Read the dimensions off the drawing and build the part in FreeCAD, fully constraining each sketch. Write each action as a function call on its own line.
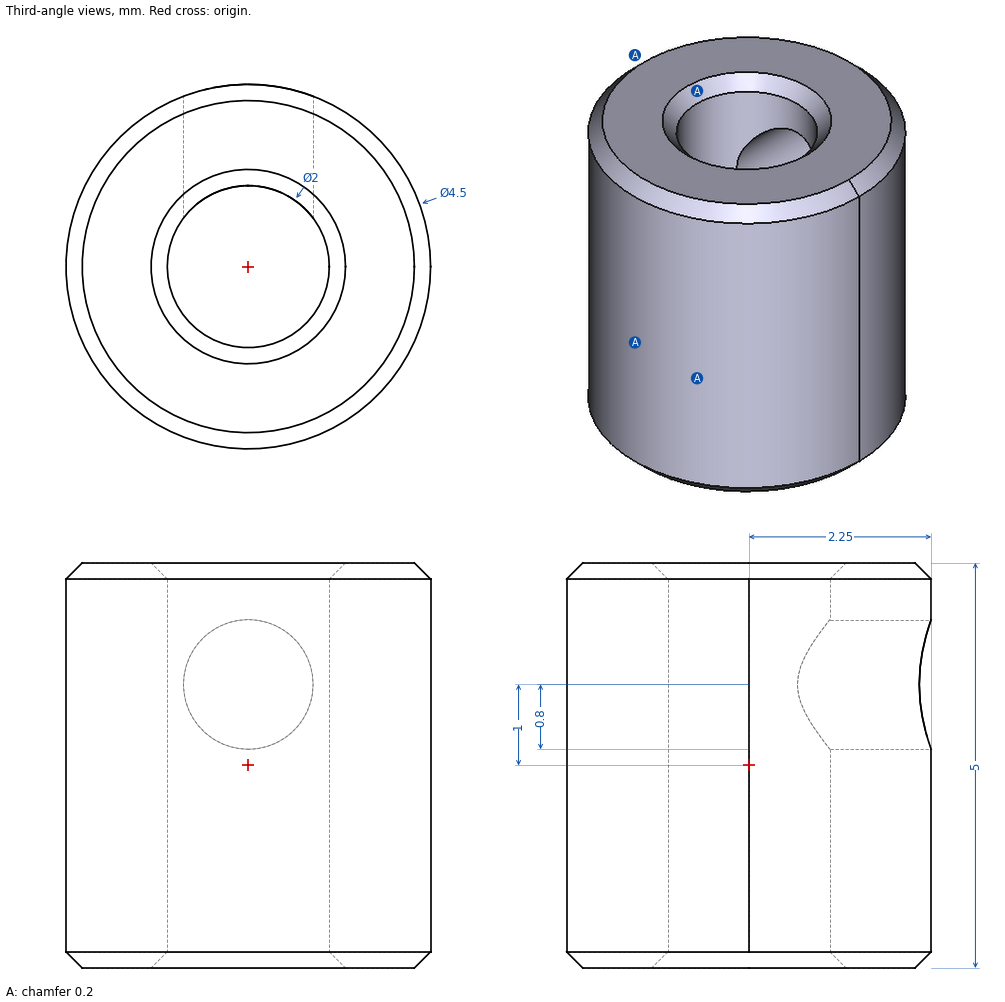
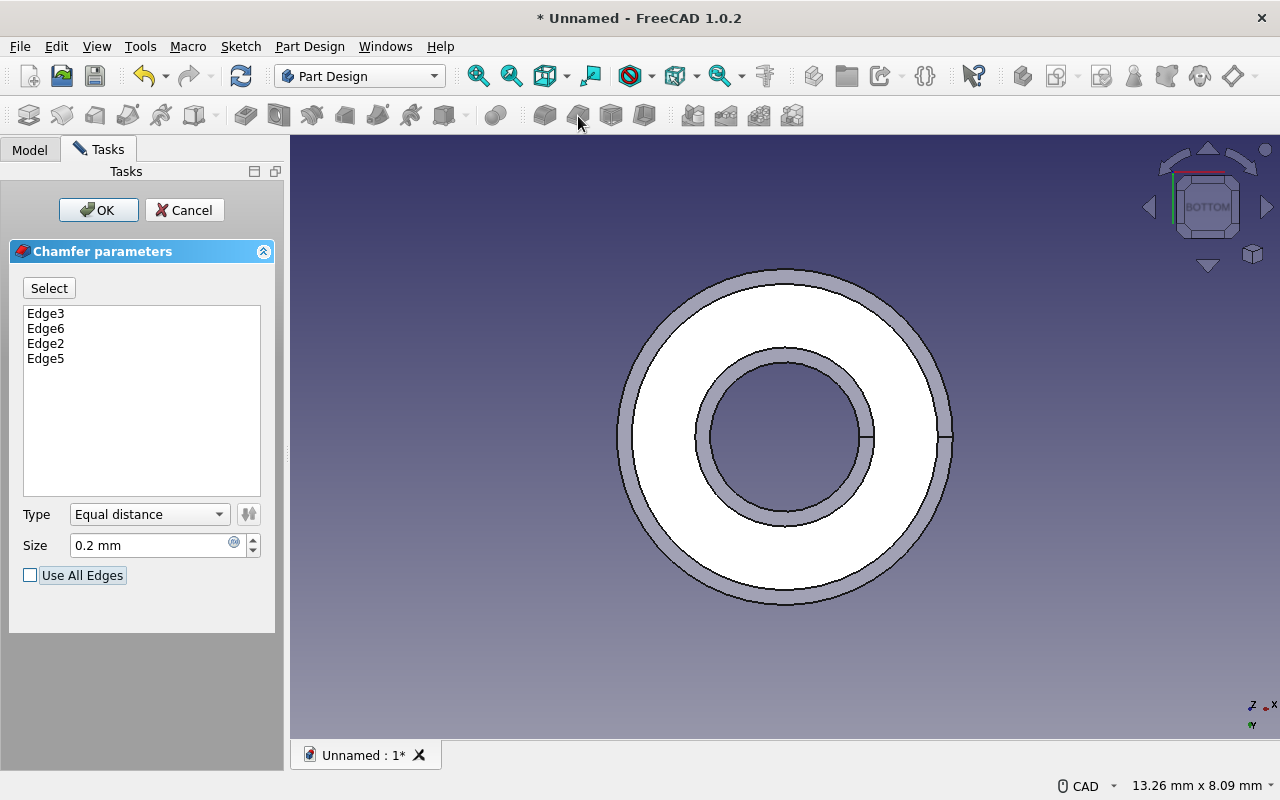
click(99, 210)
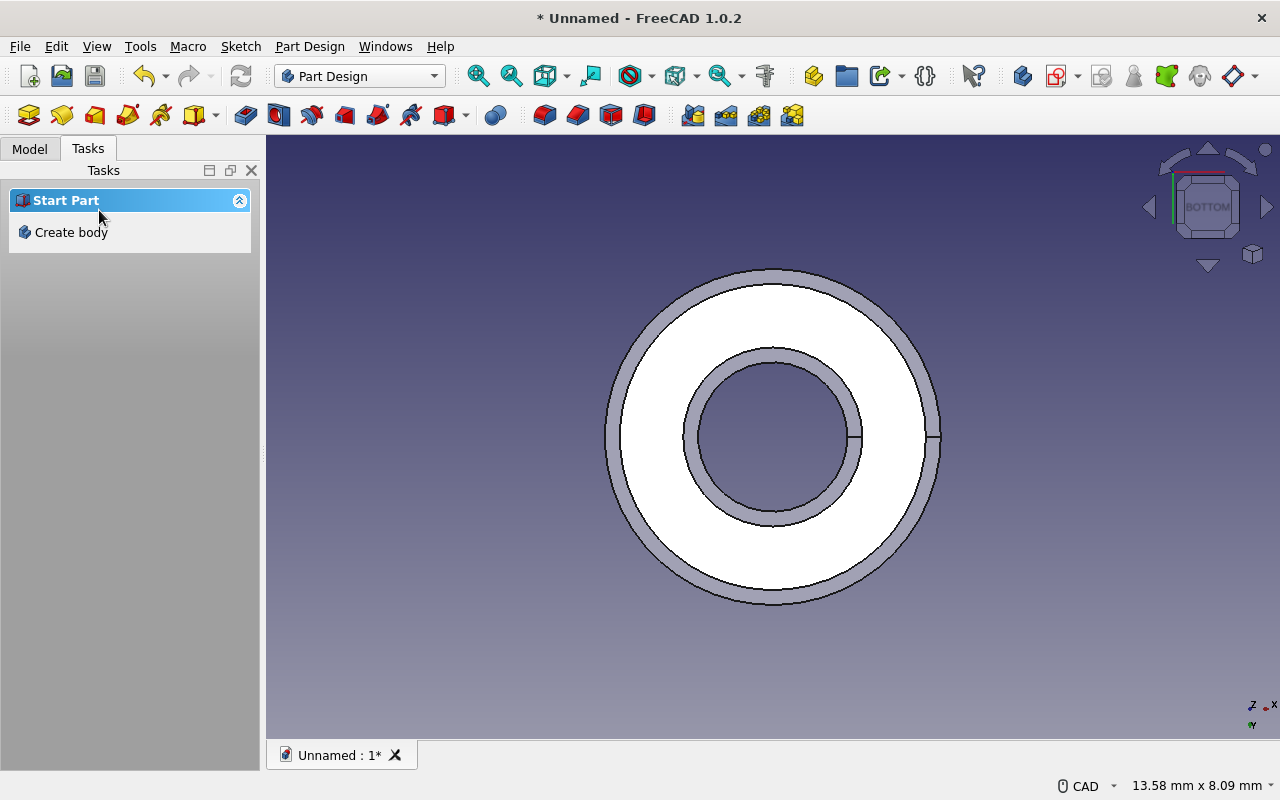
click(1056, 76)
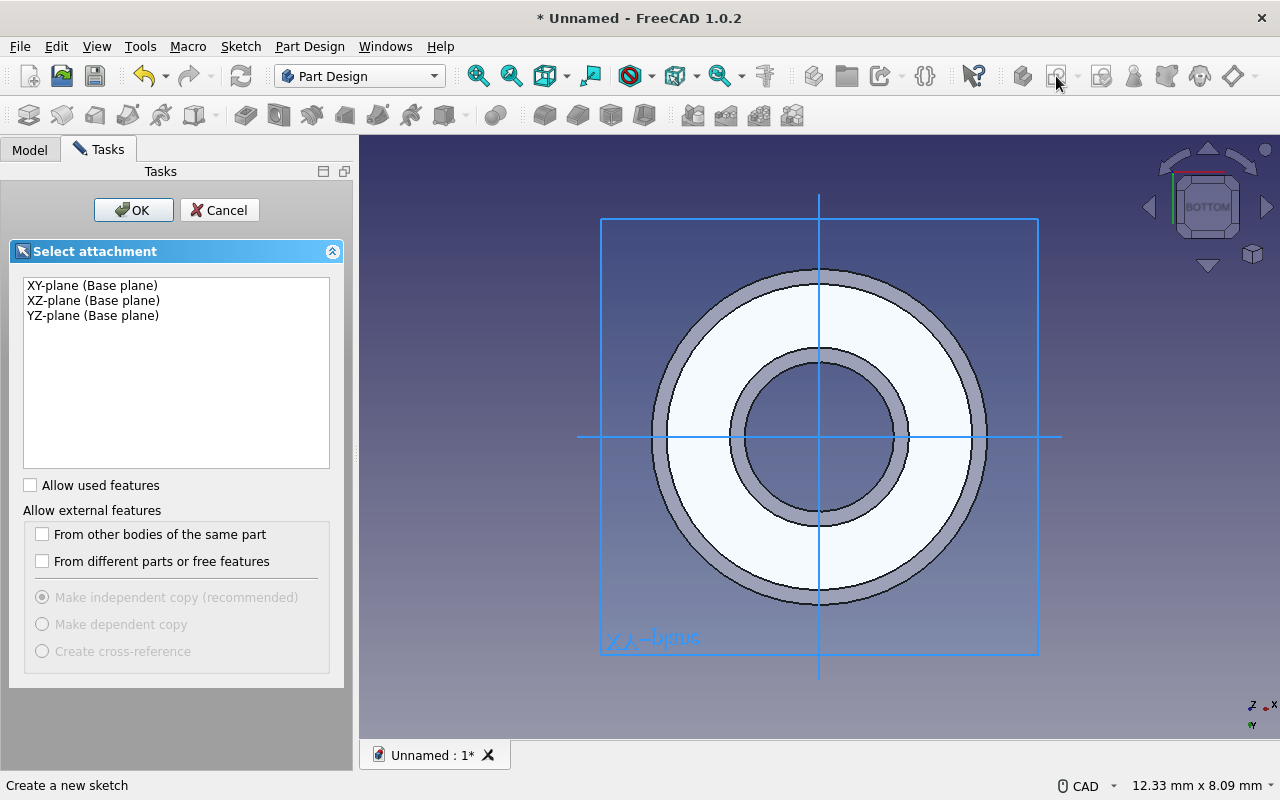
click(84, 316)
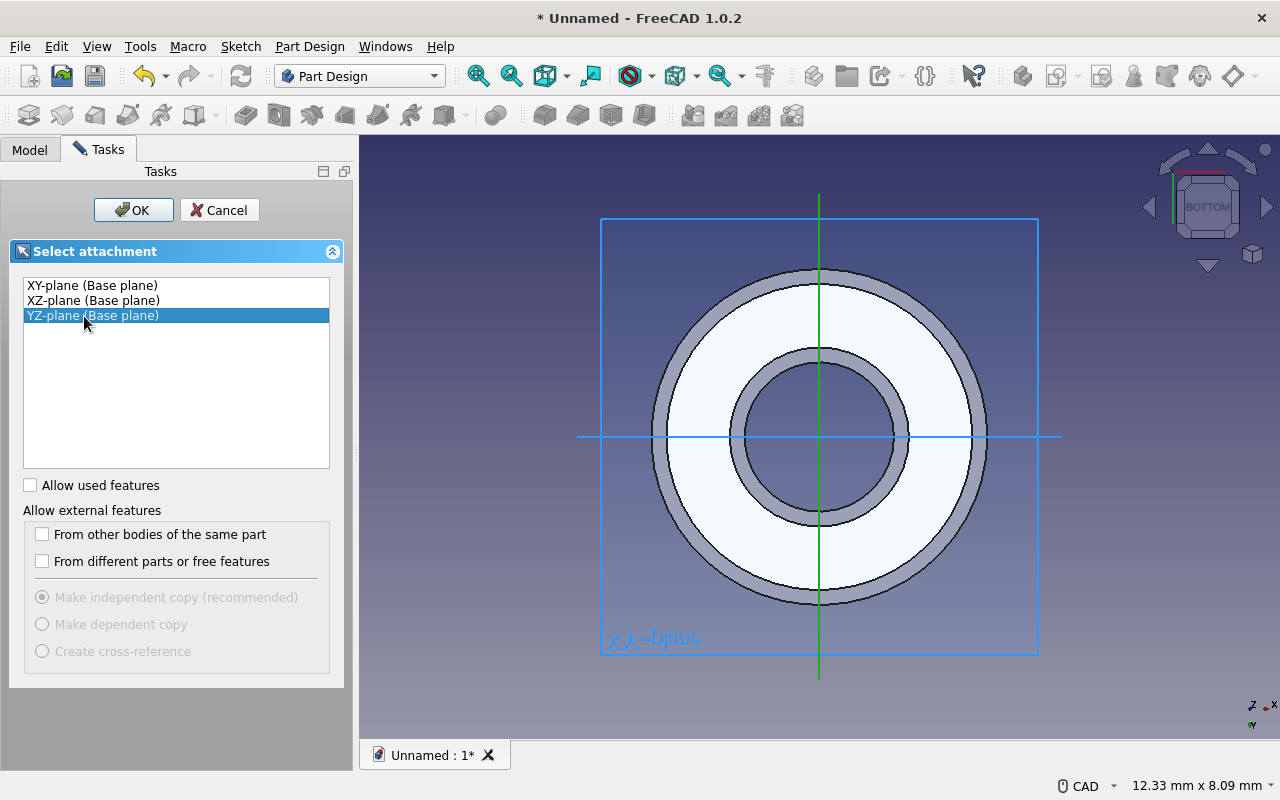
click(134, 210)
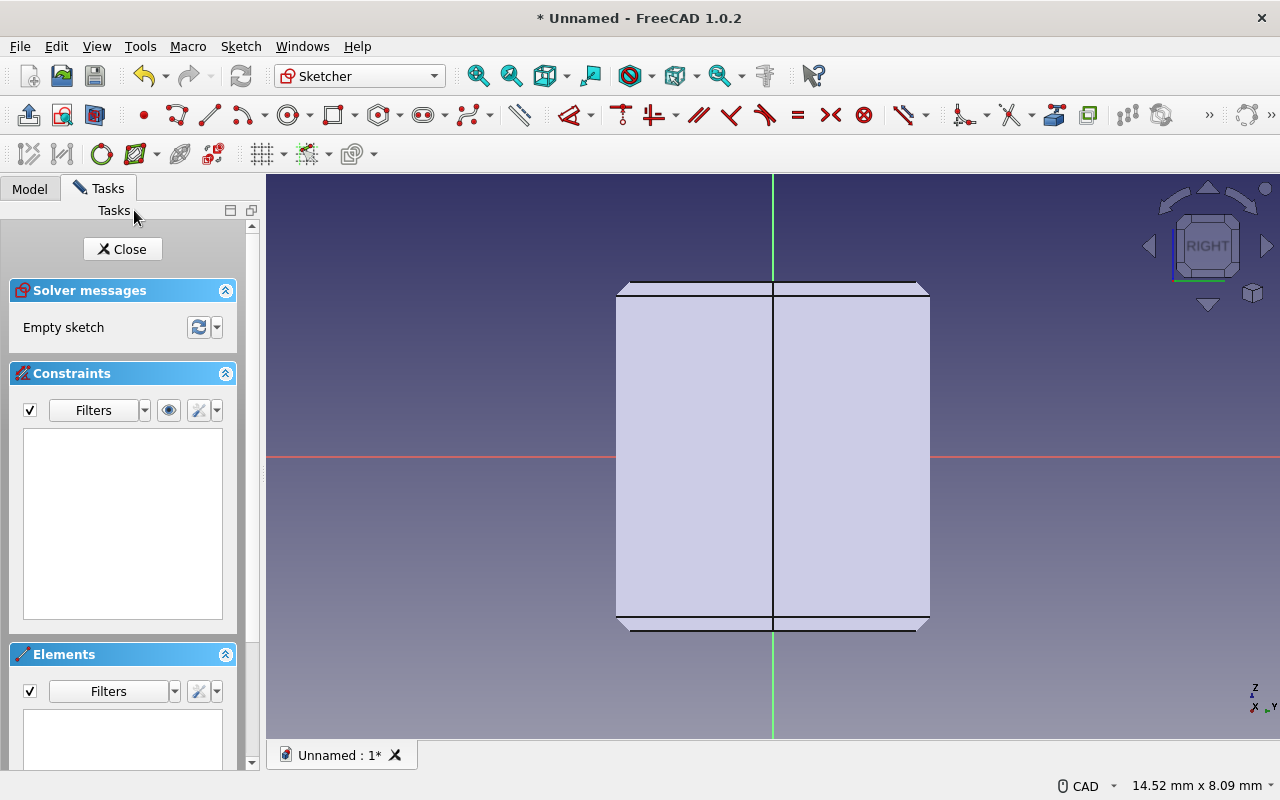
click(95, 116)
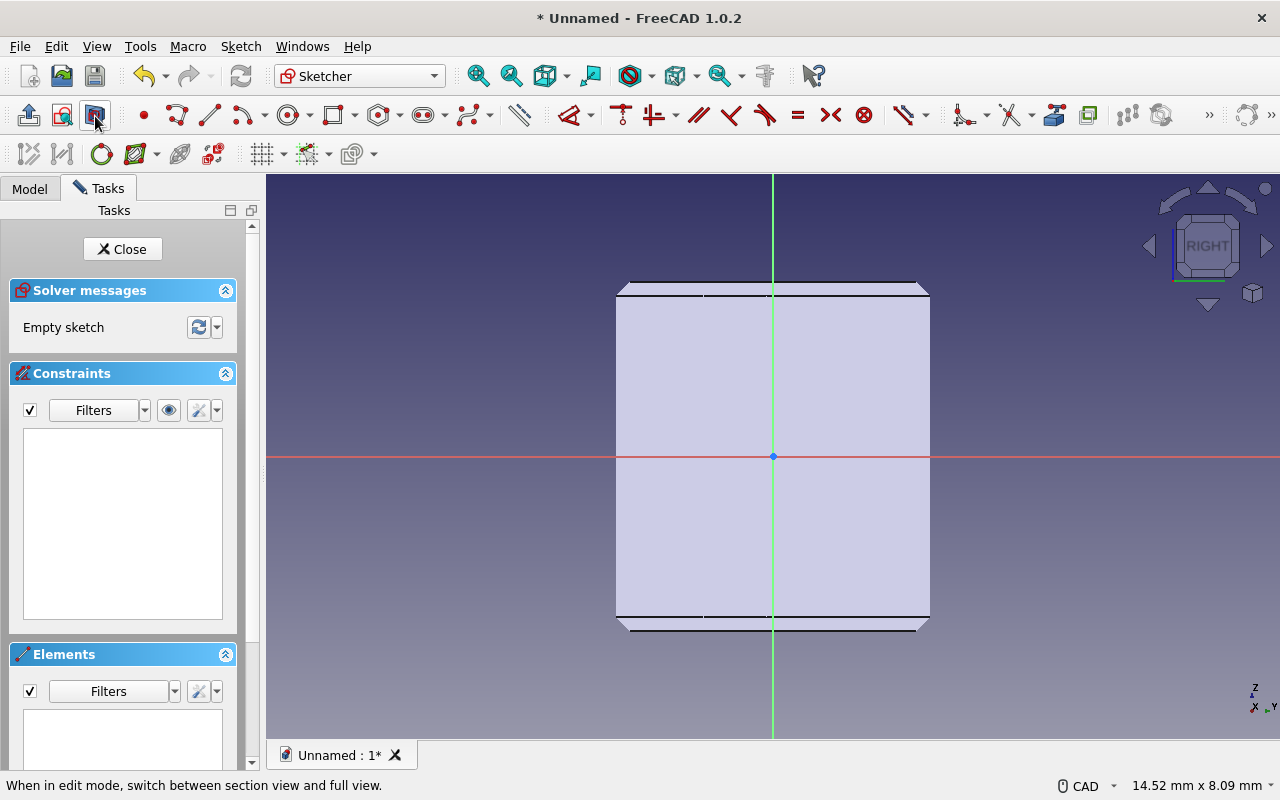
scroll(987, 401, up, 5)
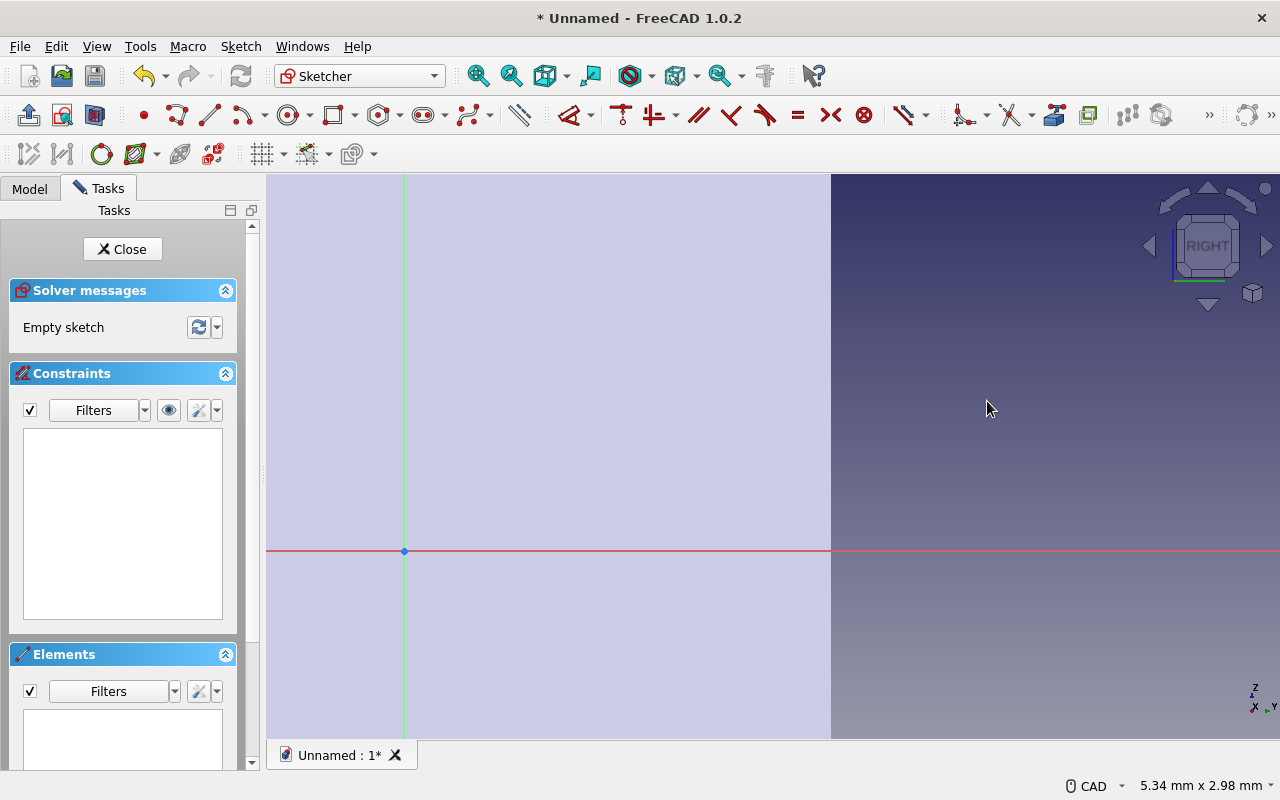
key(g)
key(r)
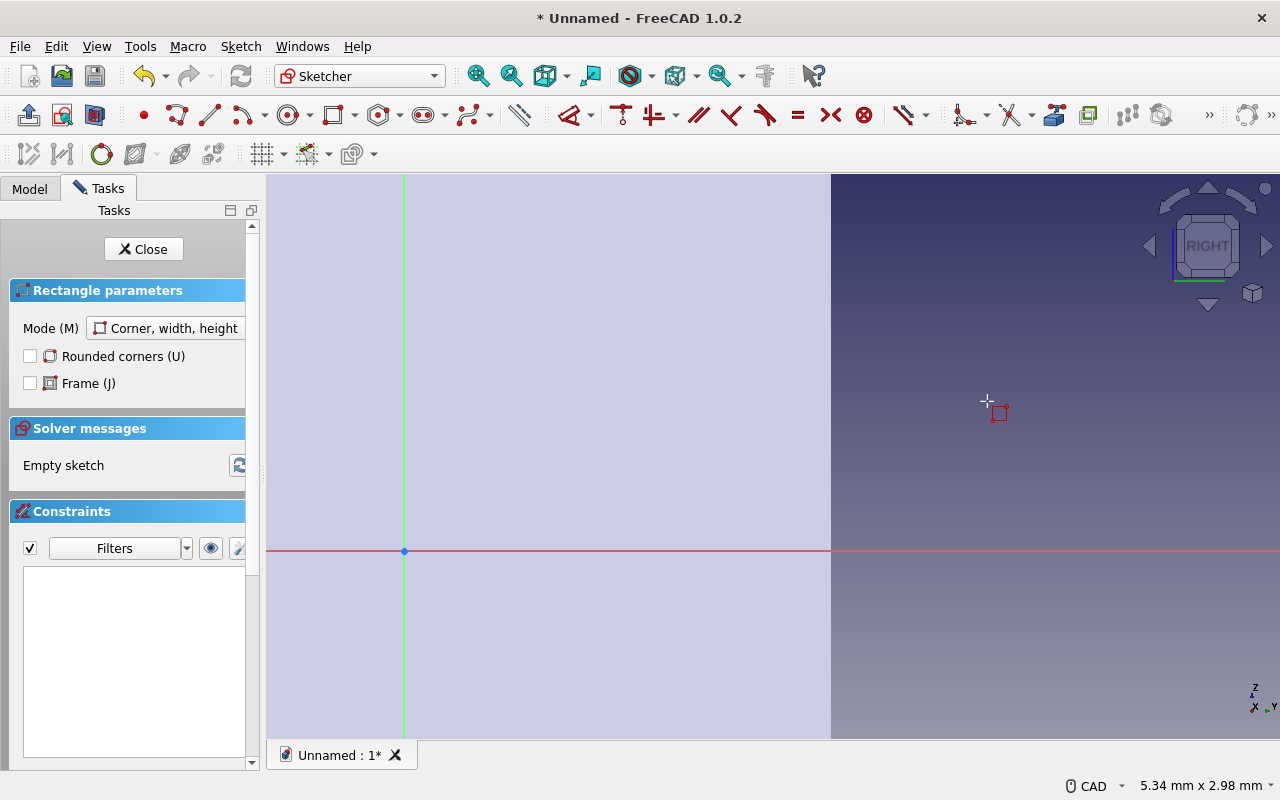
click(404, 361)
click(831, 513)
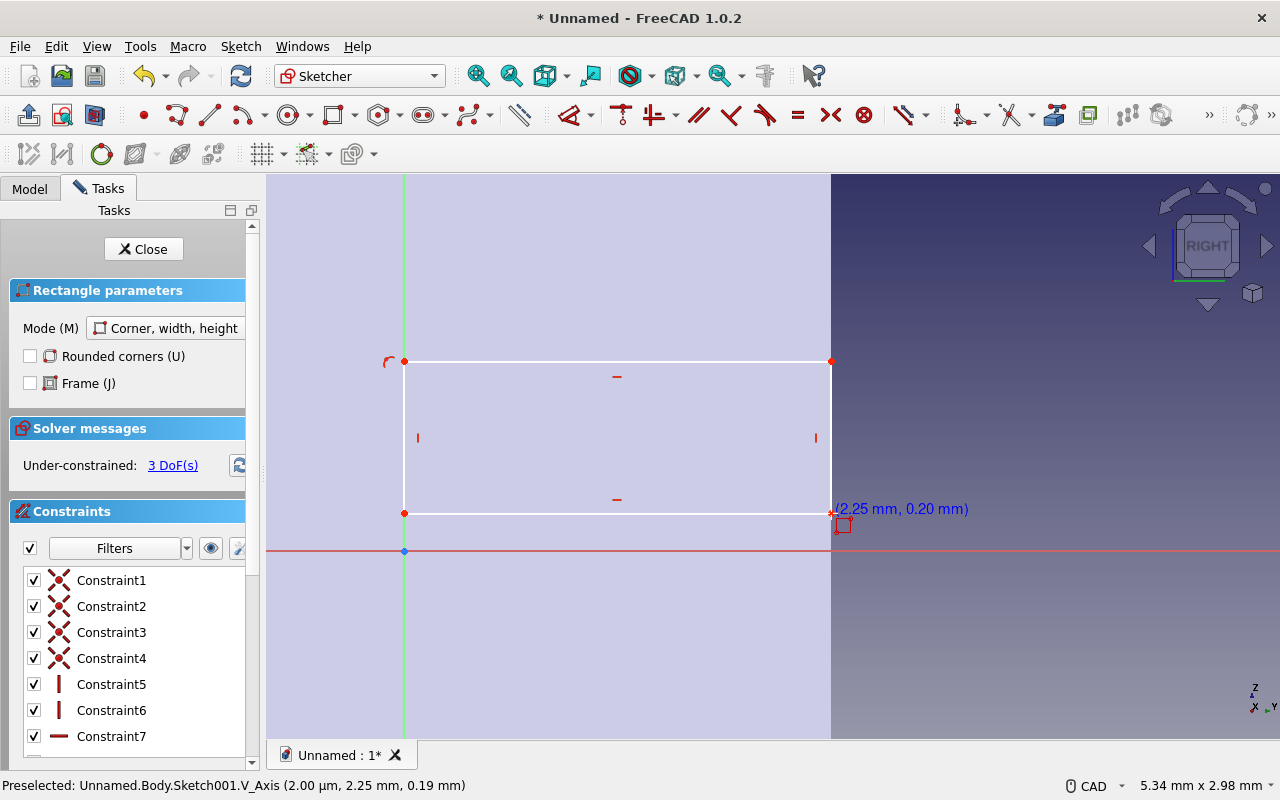
click(210, 116)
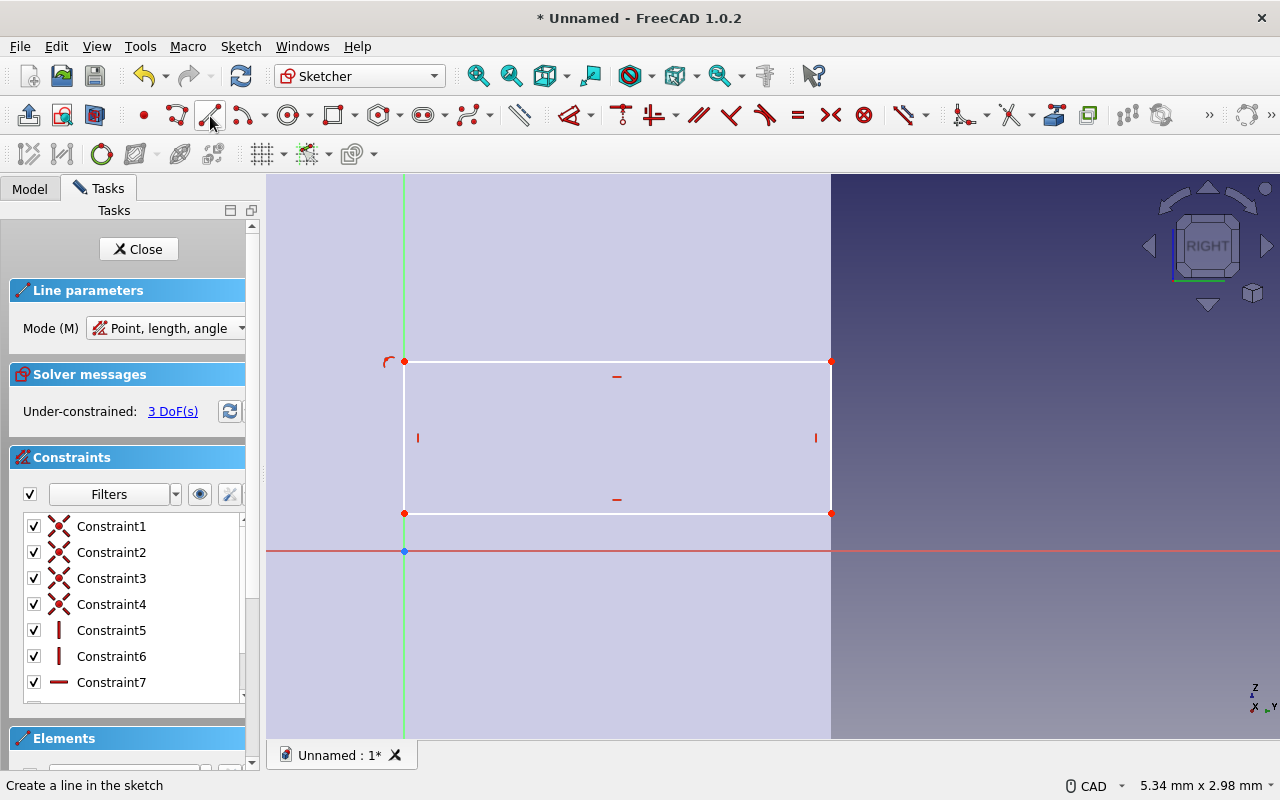
click(874, 361)
click(1002, 361)
key(Escape)